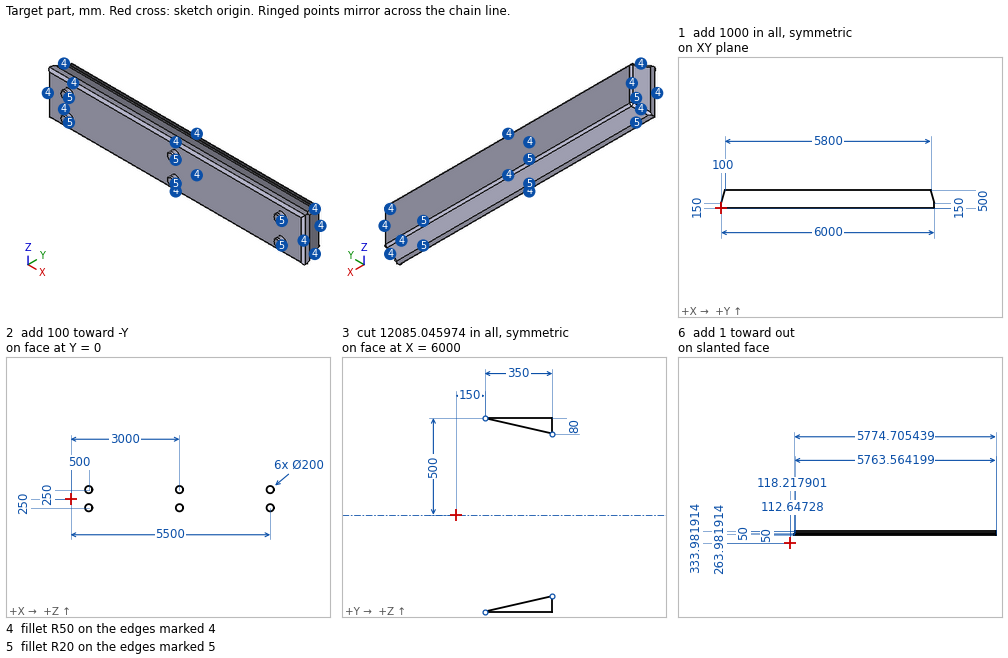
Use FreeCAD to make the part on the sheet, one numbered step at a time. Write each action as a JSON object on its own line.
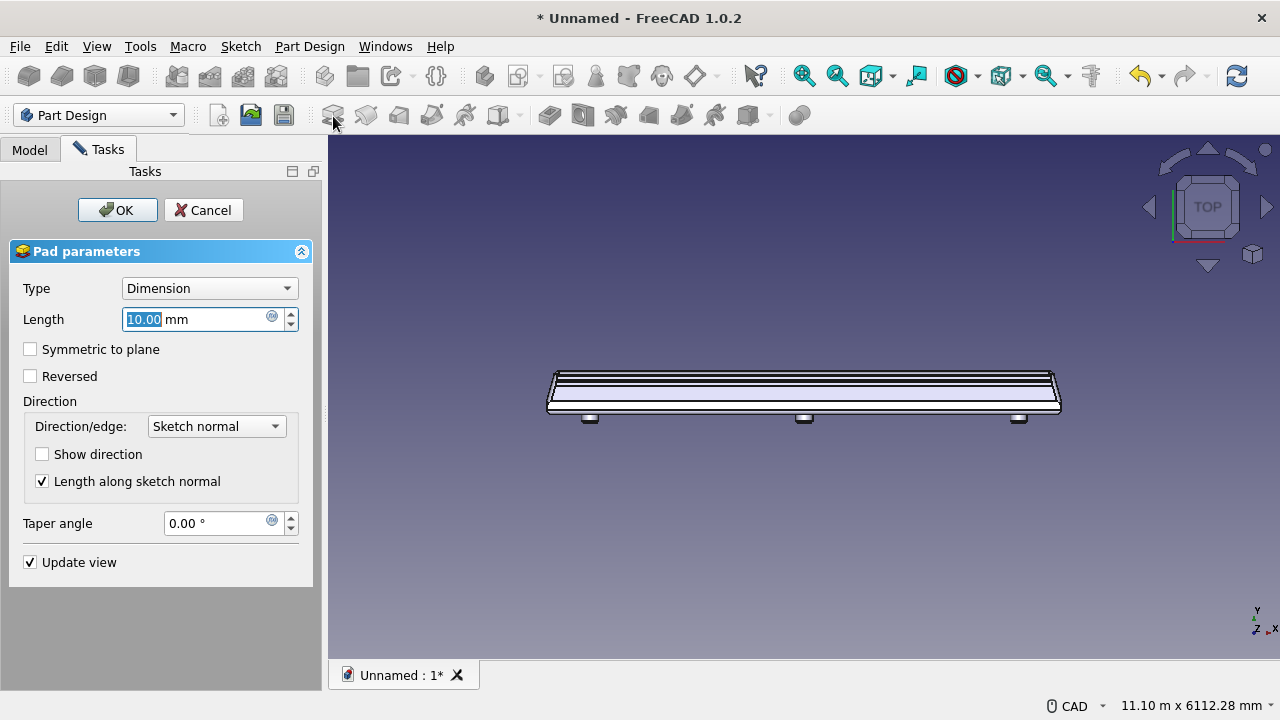
{"action": "type", "text": "1"}
{"action": "key", "text": "Tab"}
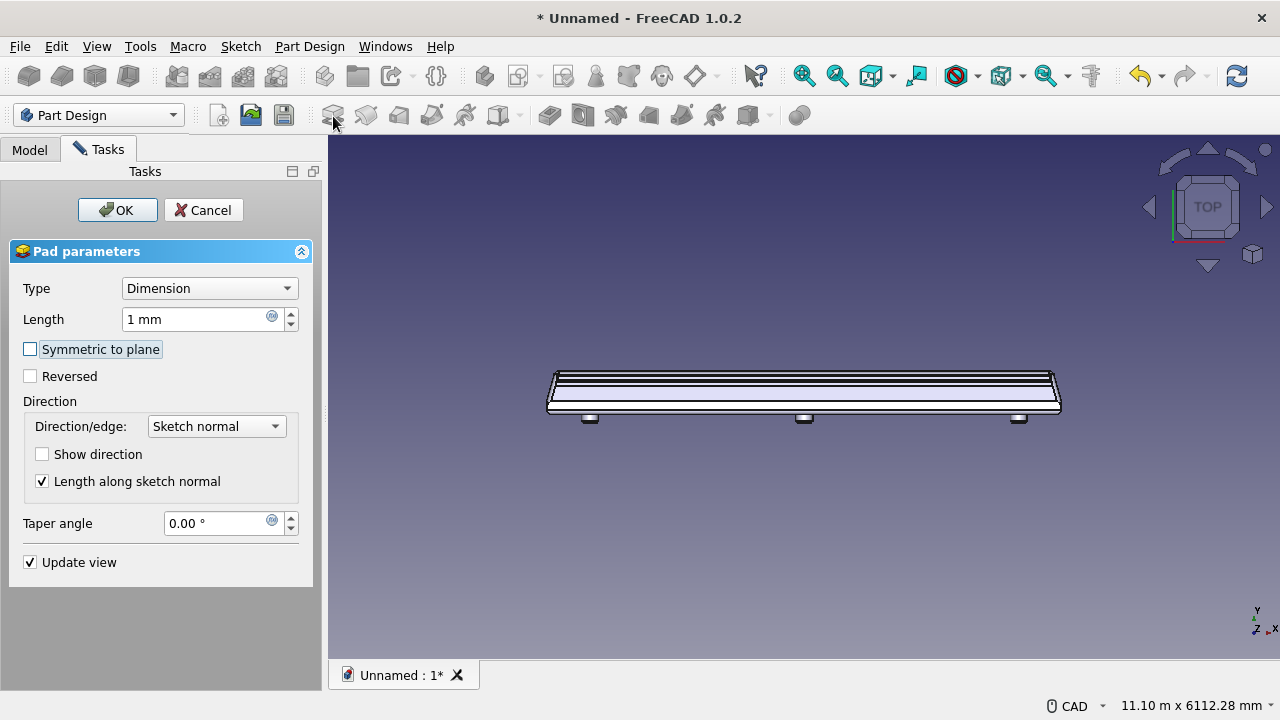
{"action": "left_click", "coordinate": [118, 210]}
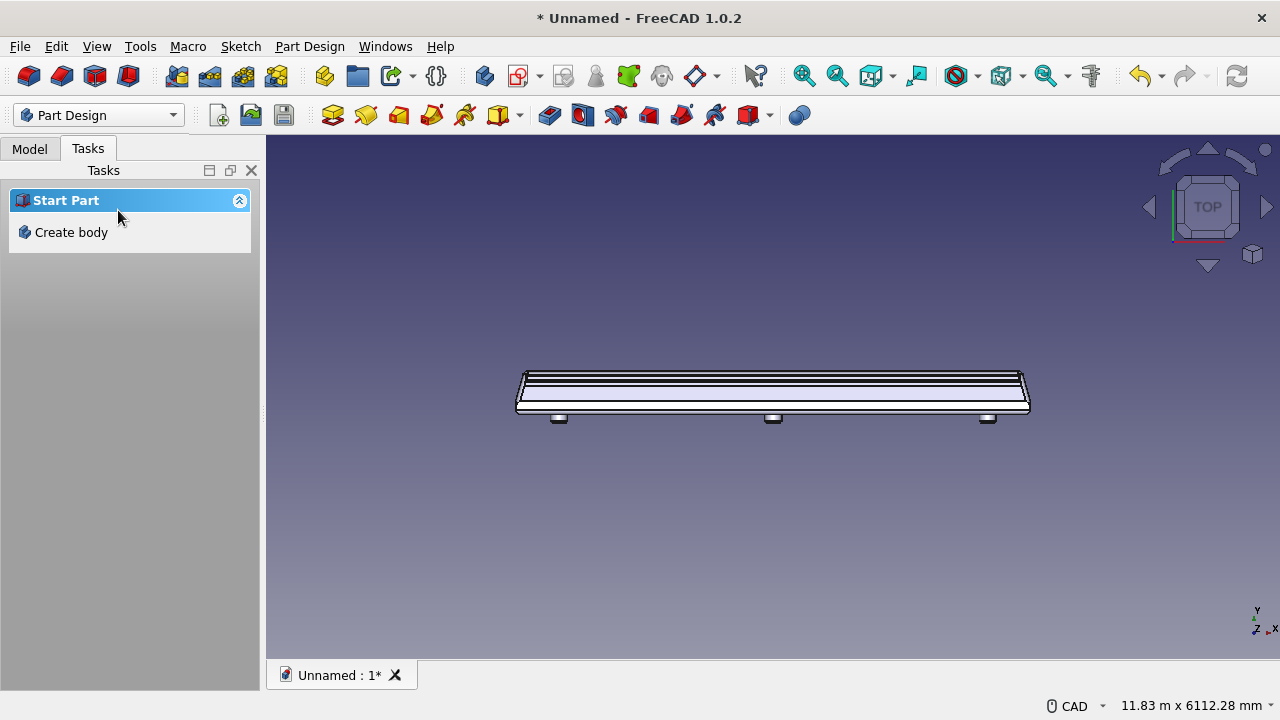
{"action": "key", "text": "0"}